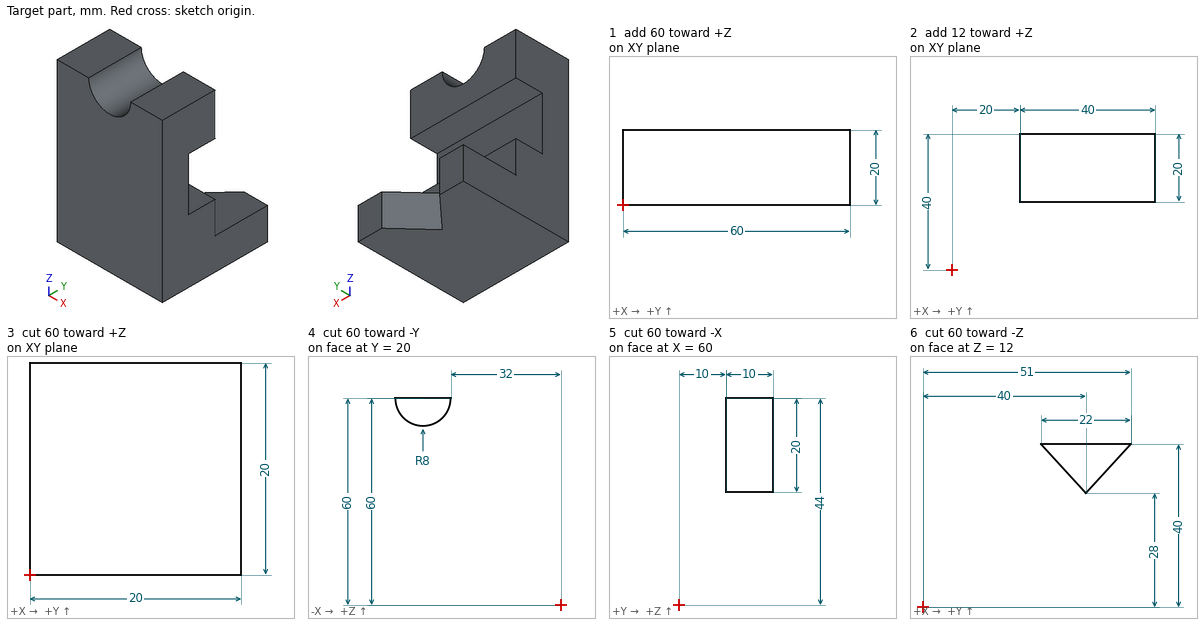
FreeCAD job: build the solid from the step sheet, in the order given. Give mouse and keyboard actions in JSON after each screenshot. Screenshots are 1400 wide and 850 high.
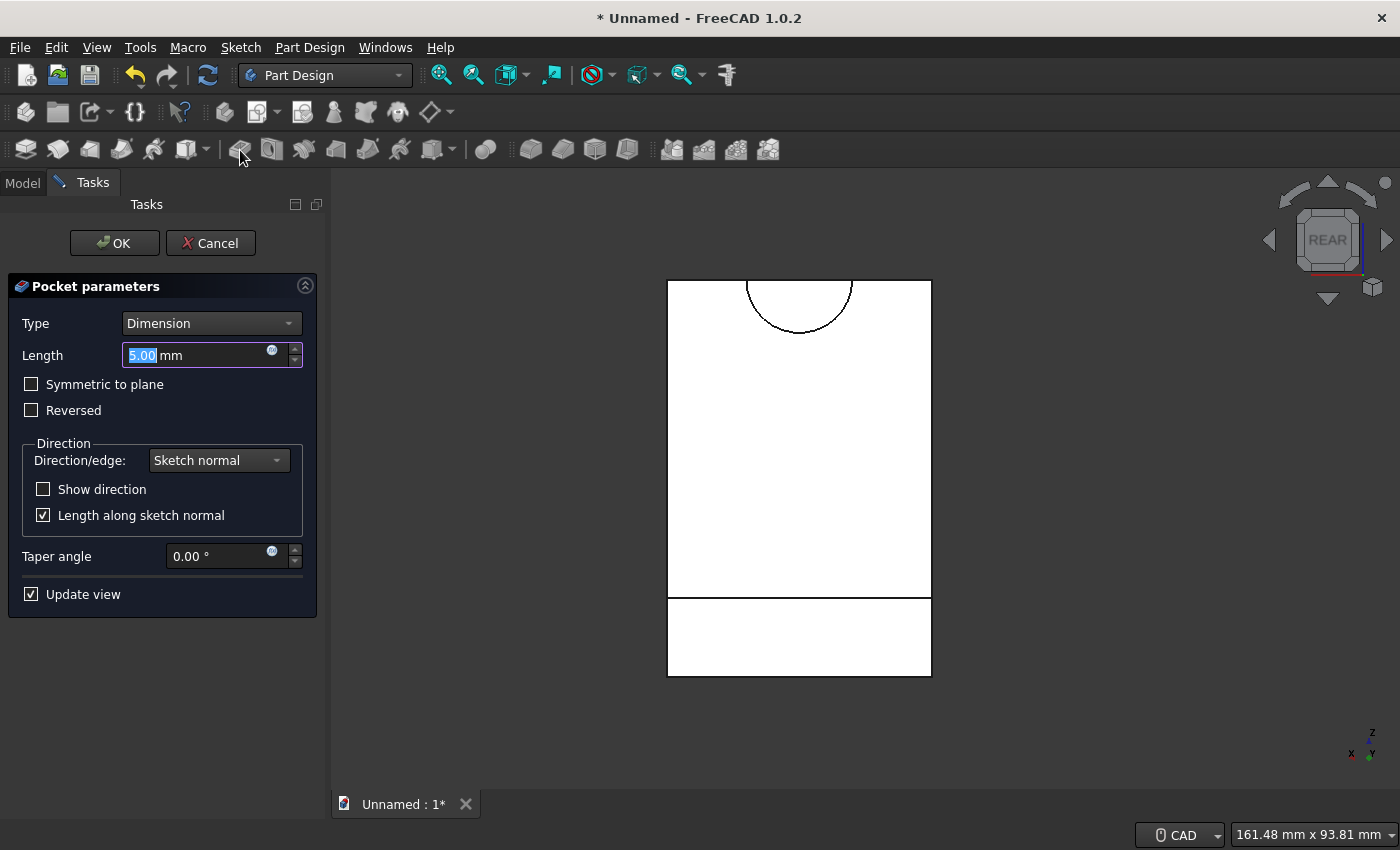
{"action": "type", "text": "60"}
{"action": "key", "text": "Tab"}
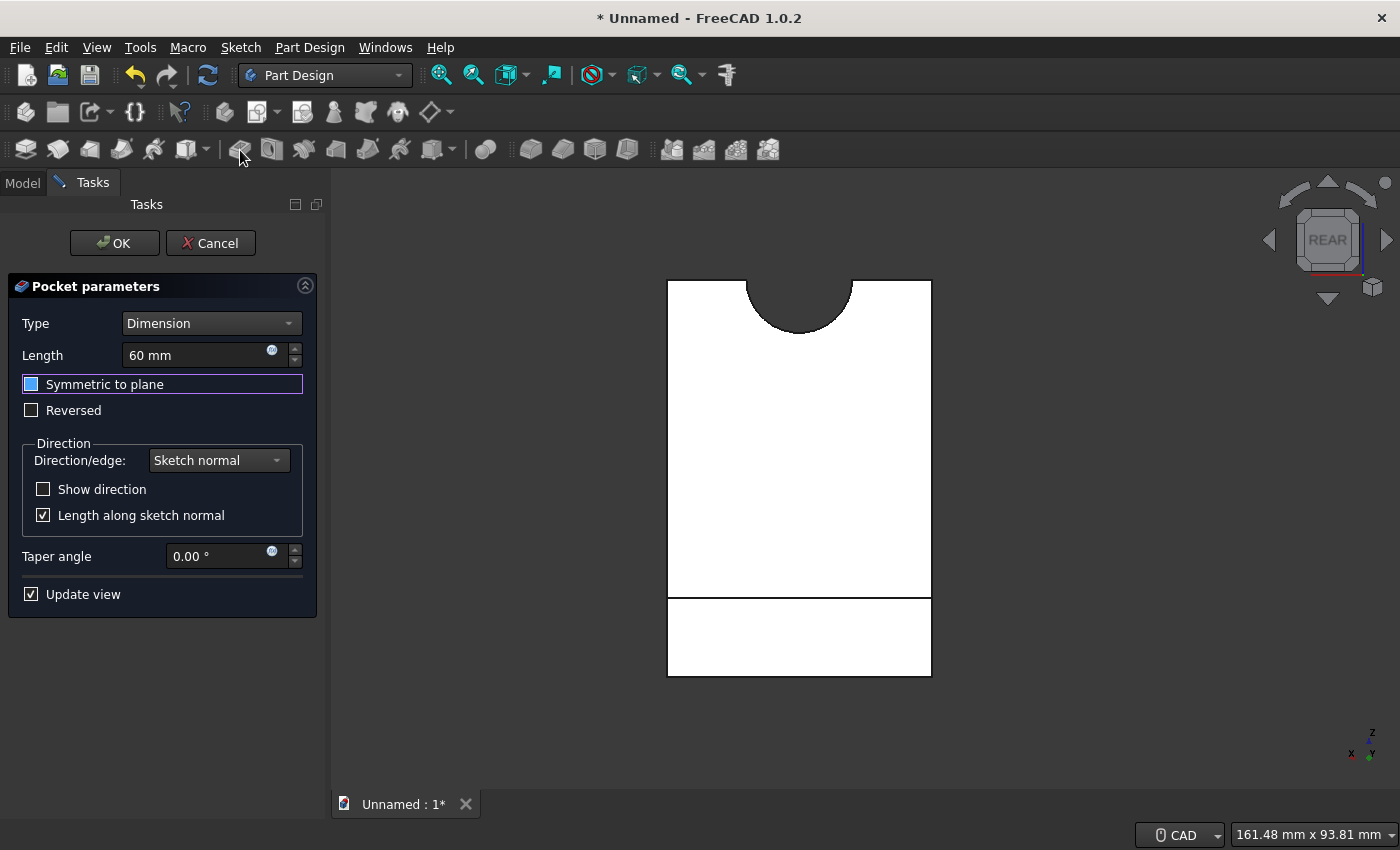
{"action": "left_click", "coordinate": [115, 243]}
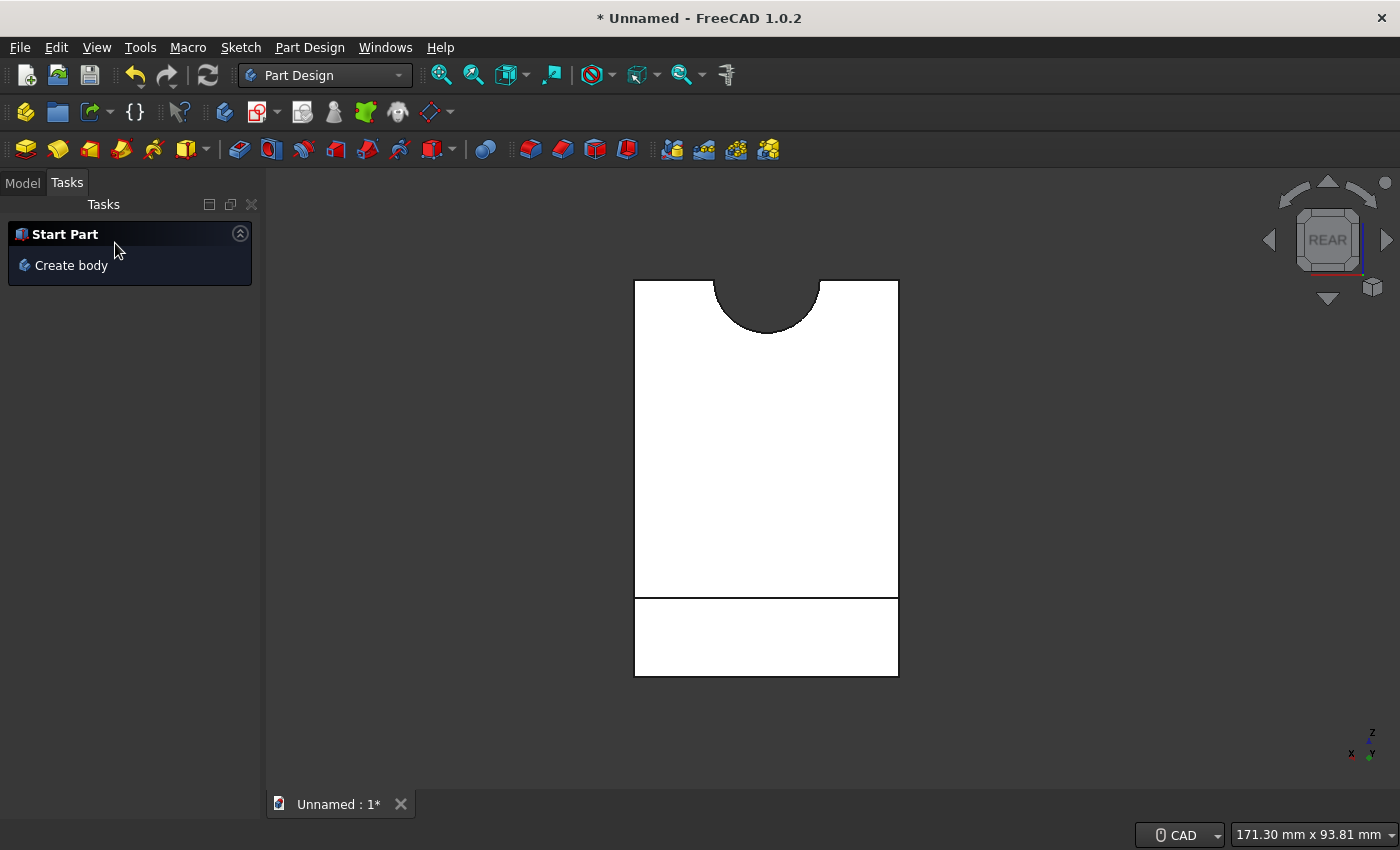
{"action": "key", "text": "0"}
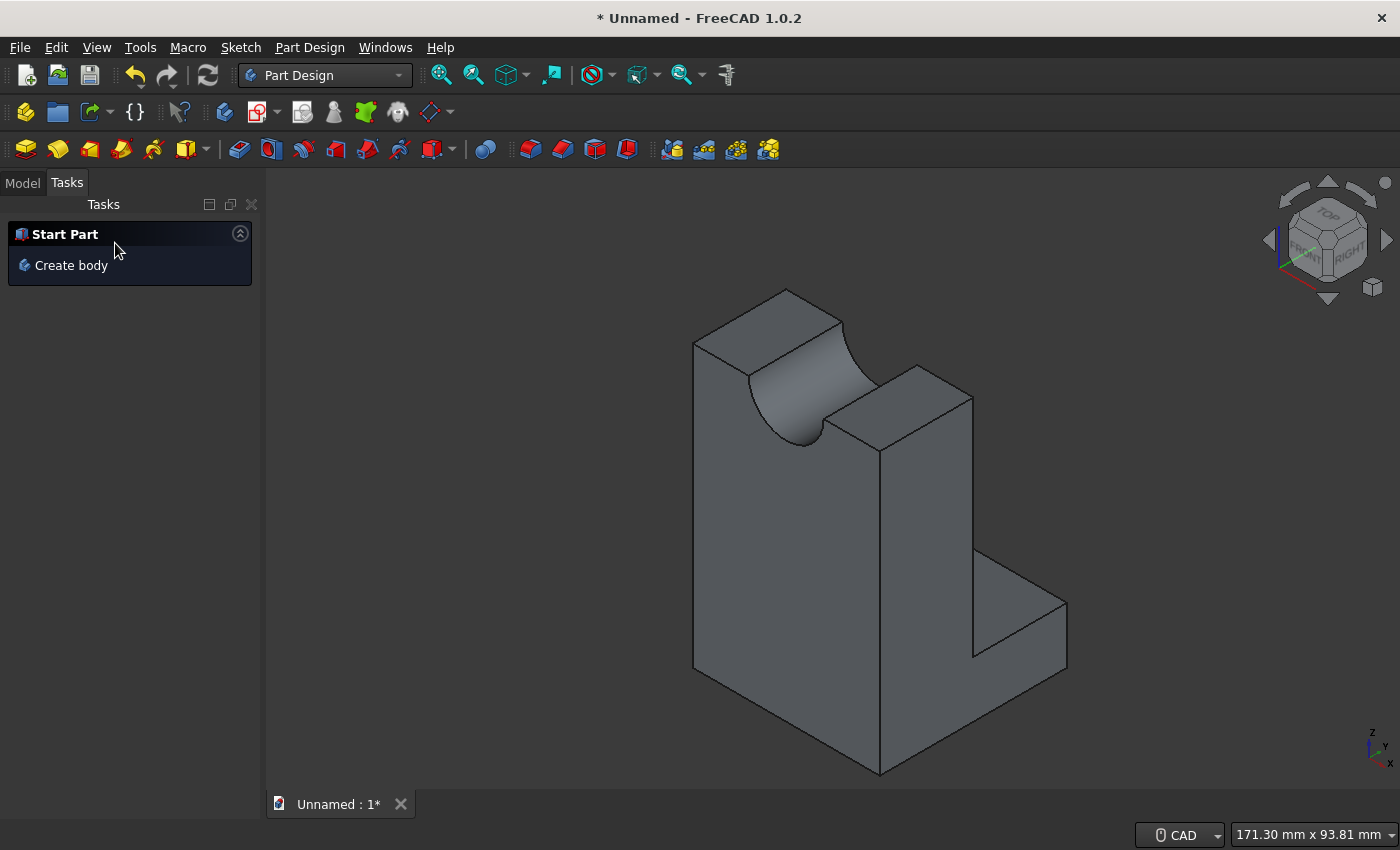
{"action": "left_click", "coordinate": [920, 497]}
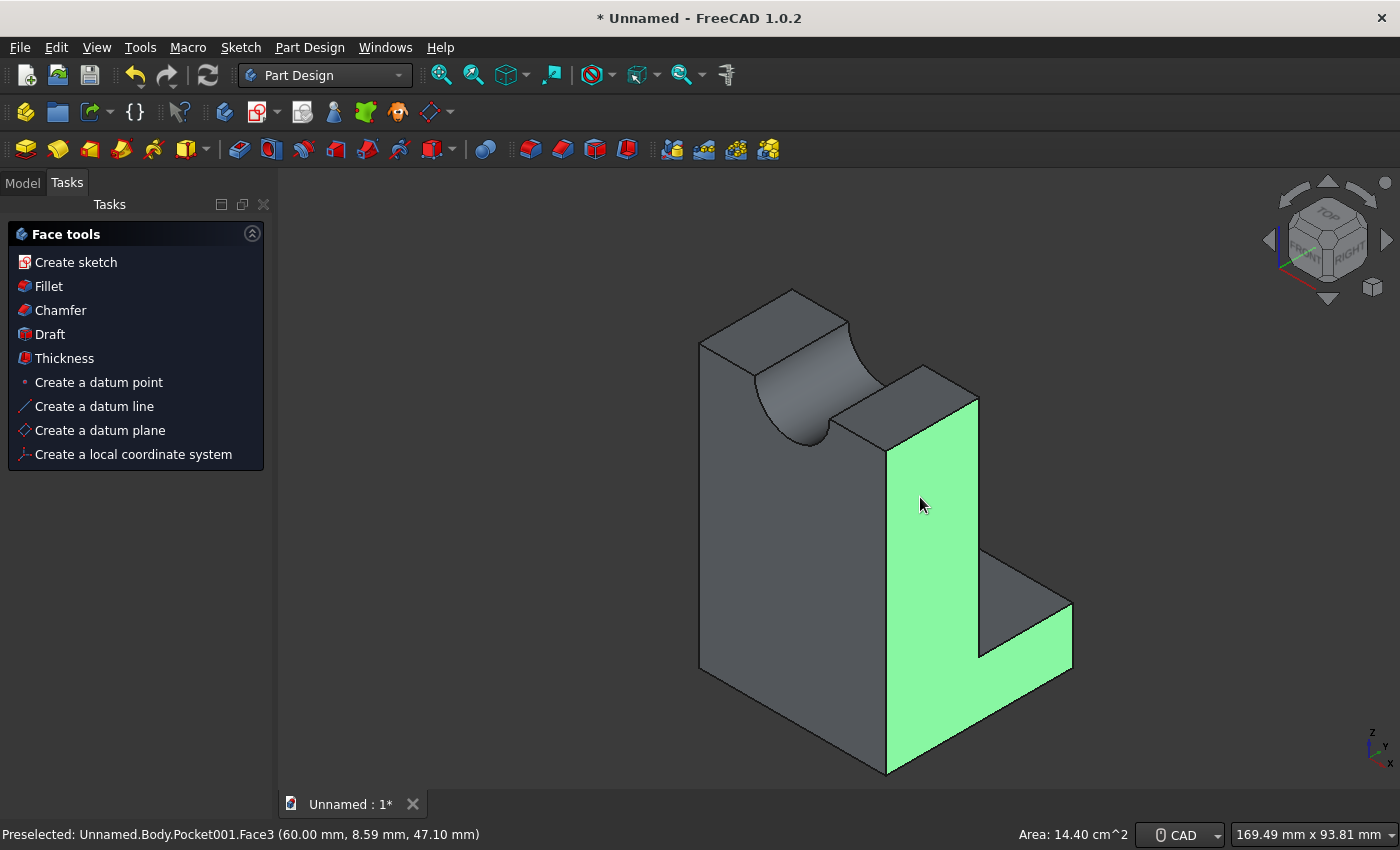
{"action": "left_click", "coordinate": [258, 112]}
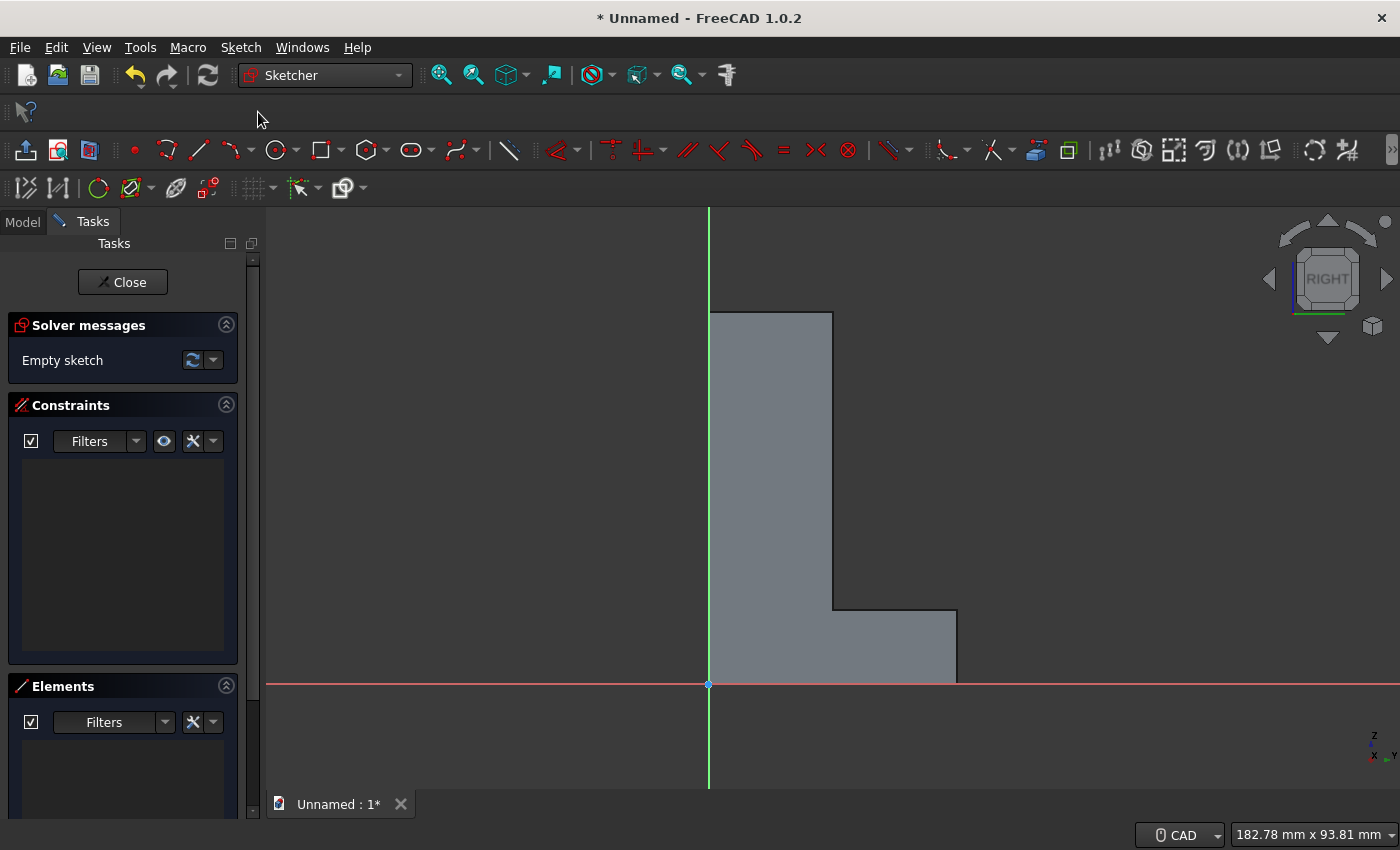
{"action": "scroll", "coordinate": [784, 649], "scroll_direction": "up", "scroll_amount": 2}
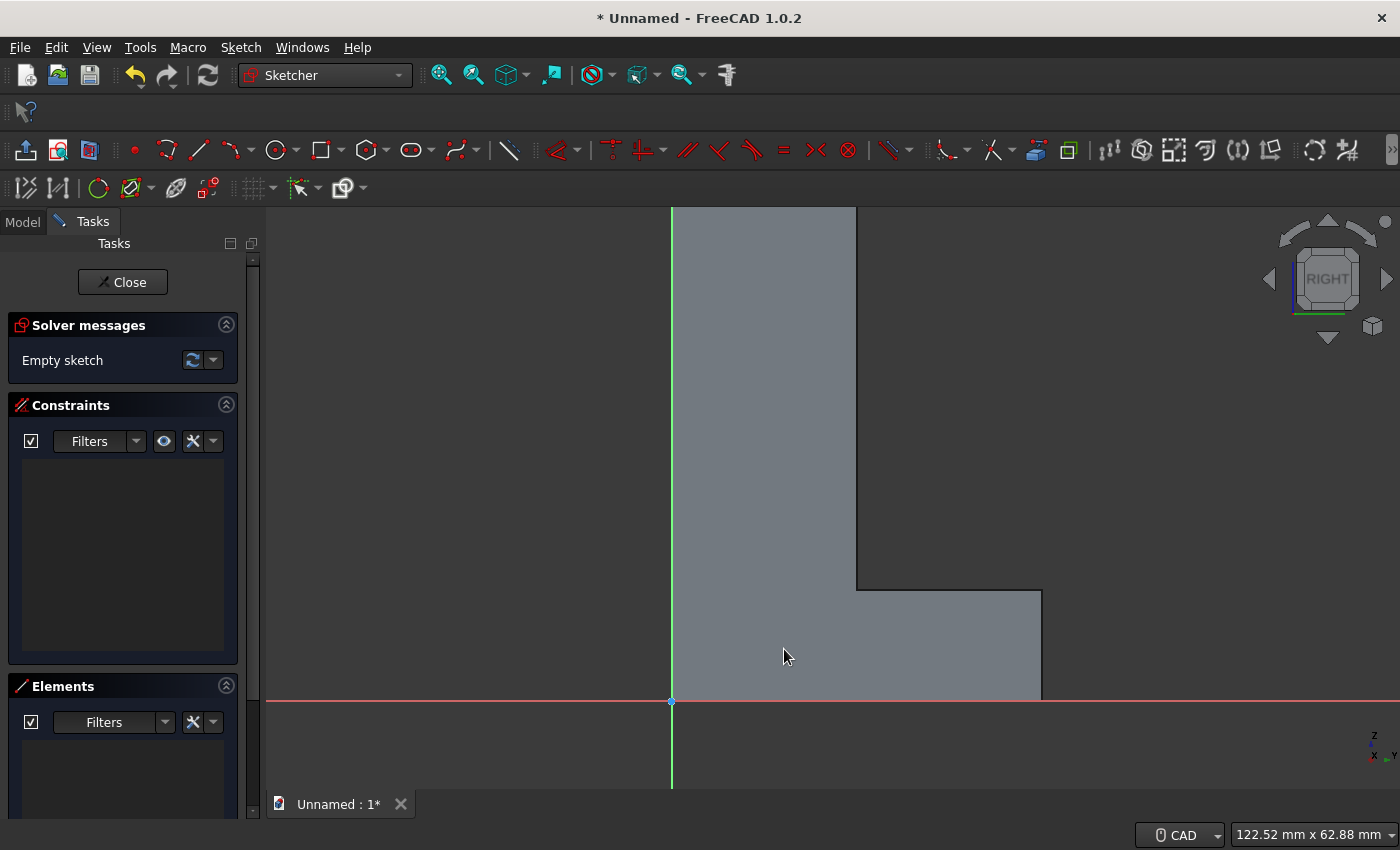
{"action": "key", "text": "g r"}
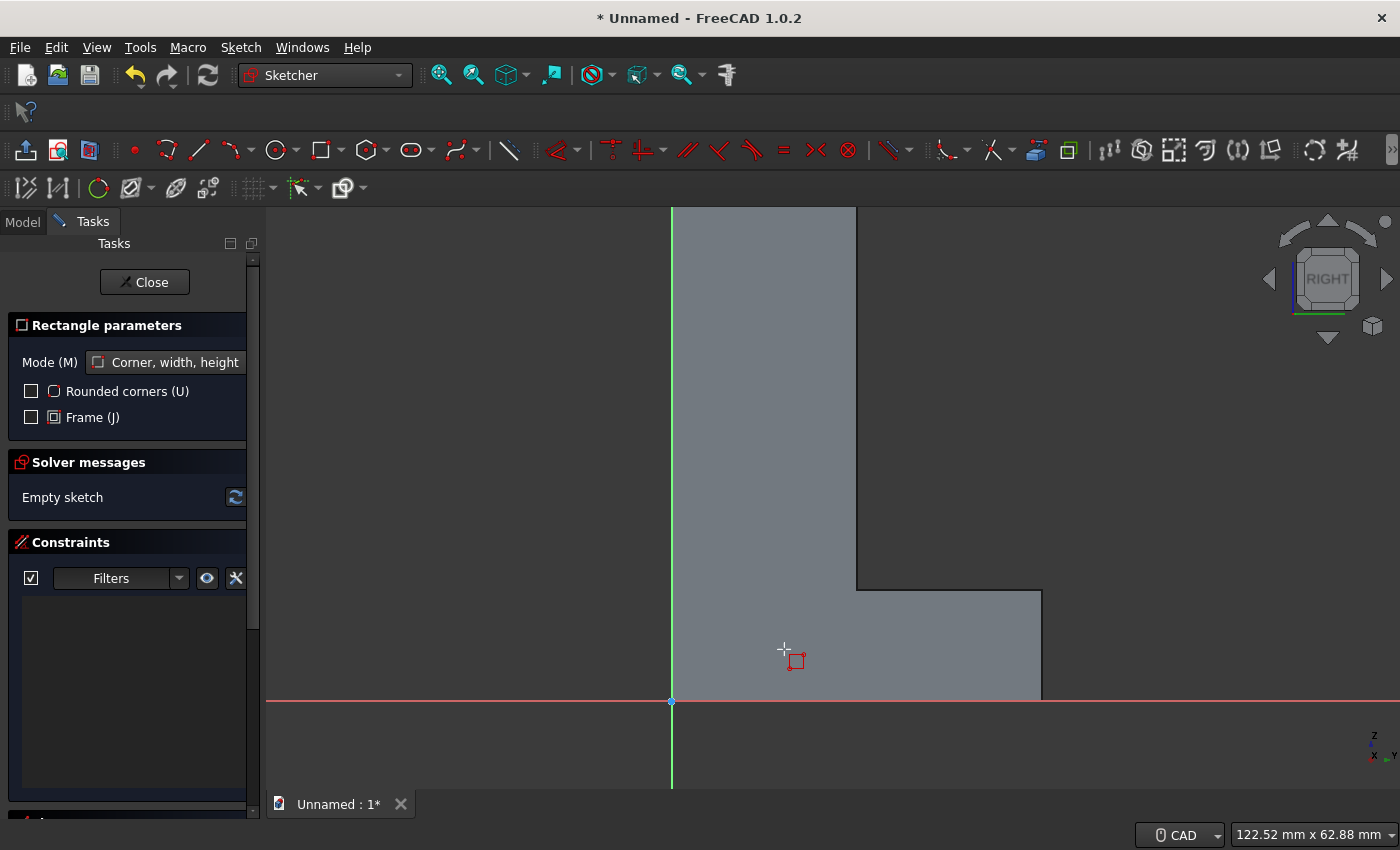
{"action": "left_click", "coordinate": [764, 294]}
{"action": "mouse_move", "coordinate": [857, 479]}